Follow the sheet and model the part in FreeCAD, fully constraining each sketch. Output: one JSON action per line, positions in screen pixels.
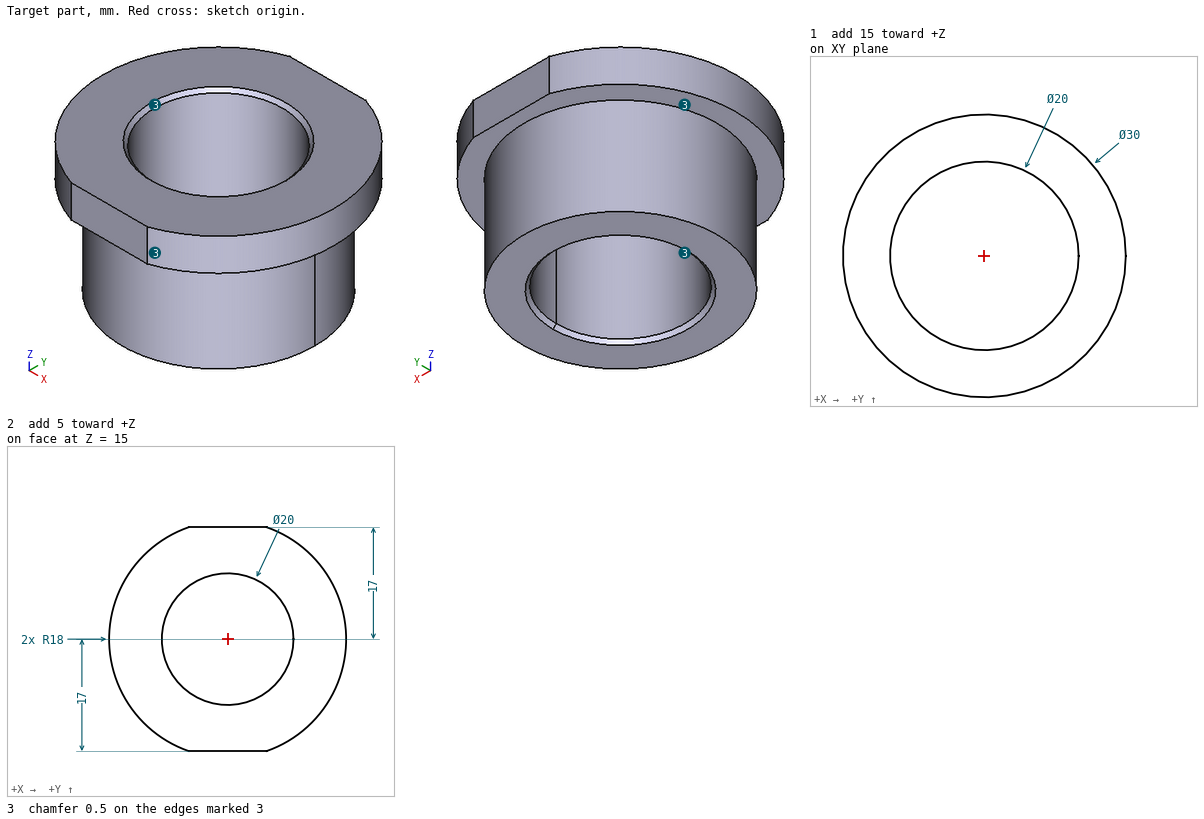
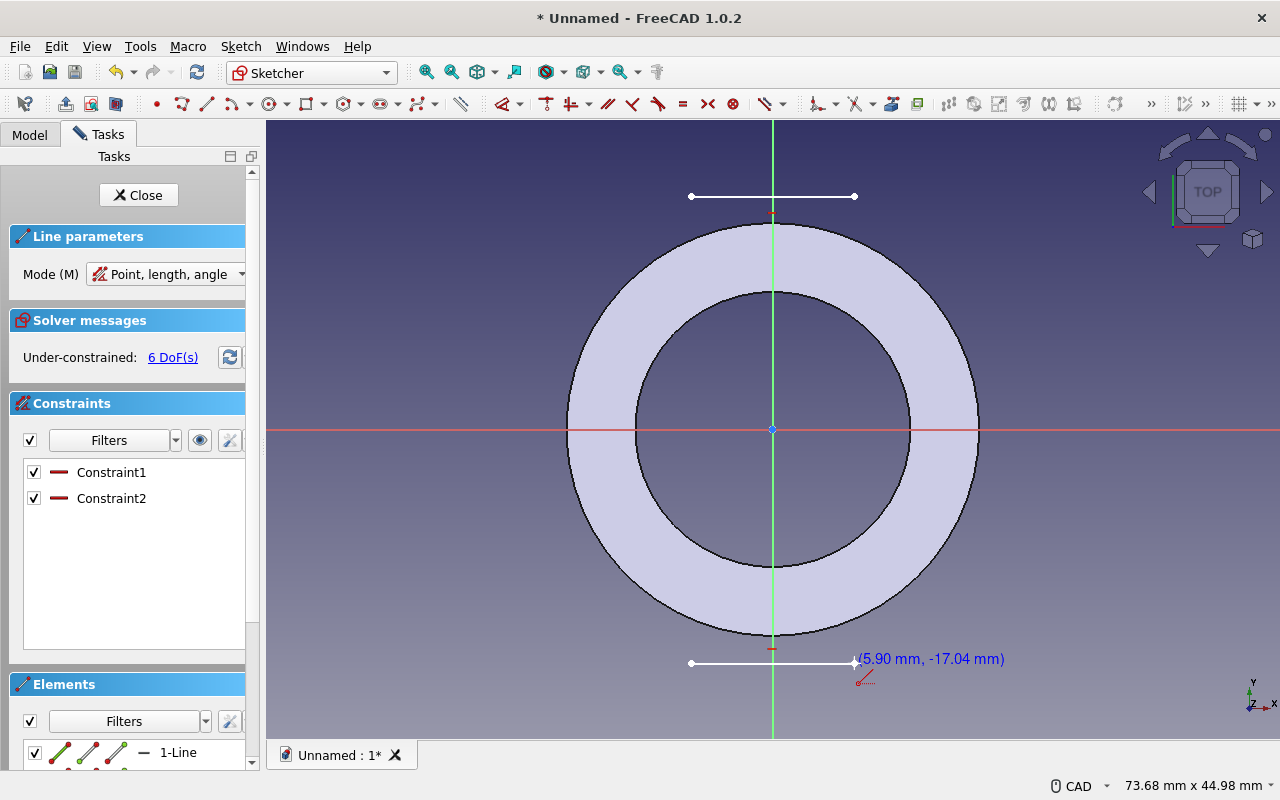
{"action": "left_click", "coordinate": [250, 104]}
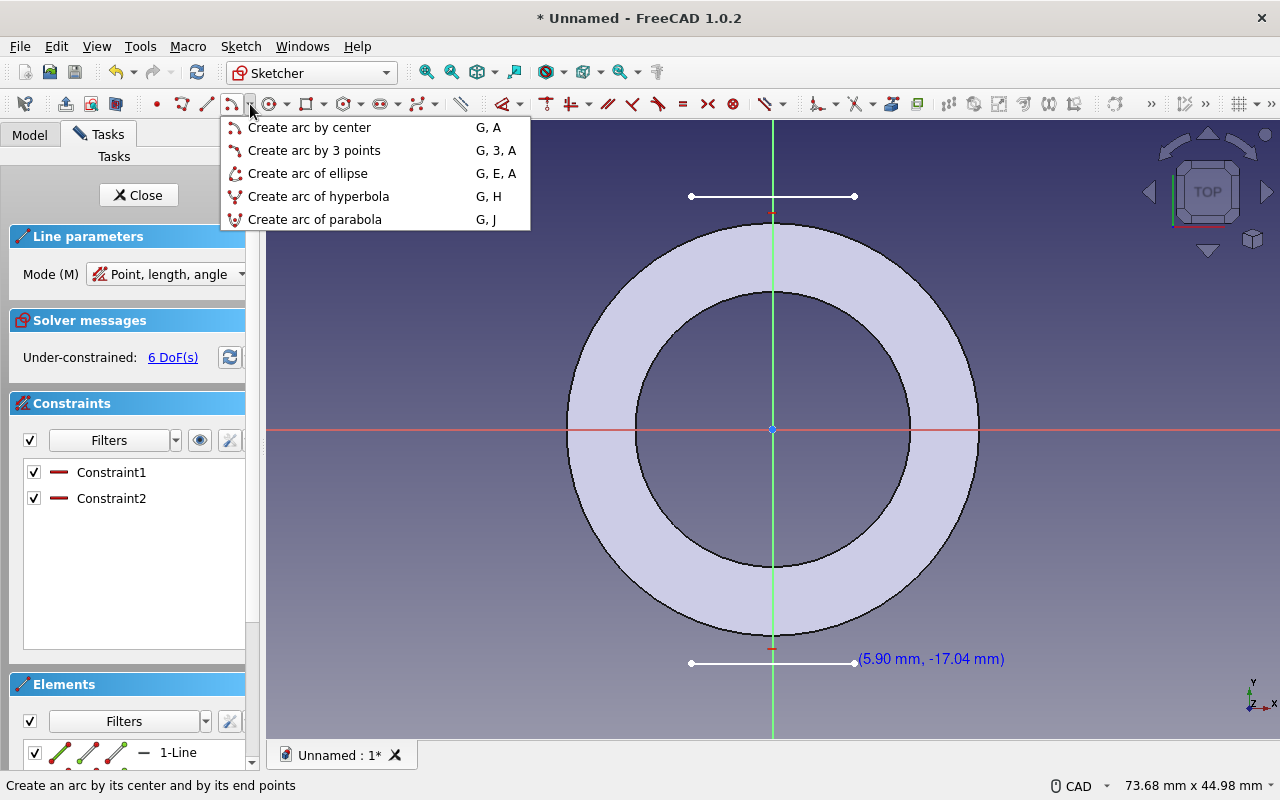
{"action": "left_click", "coordinate": [376, 150]}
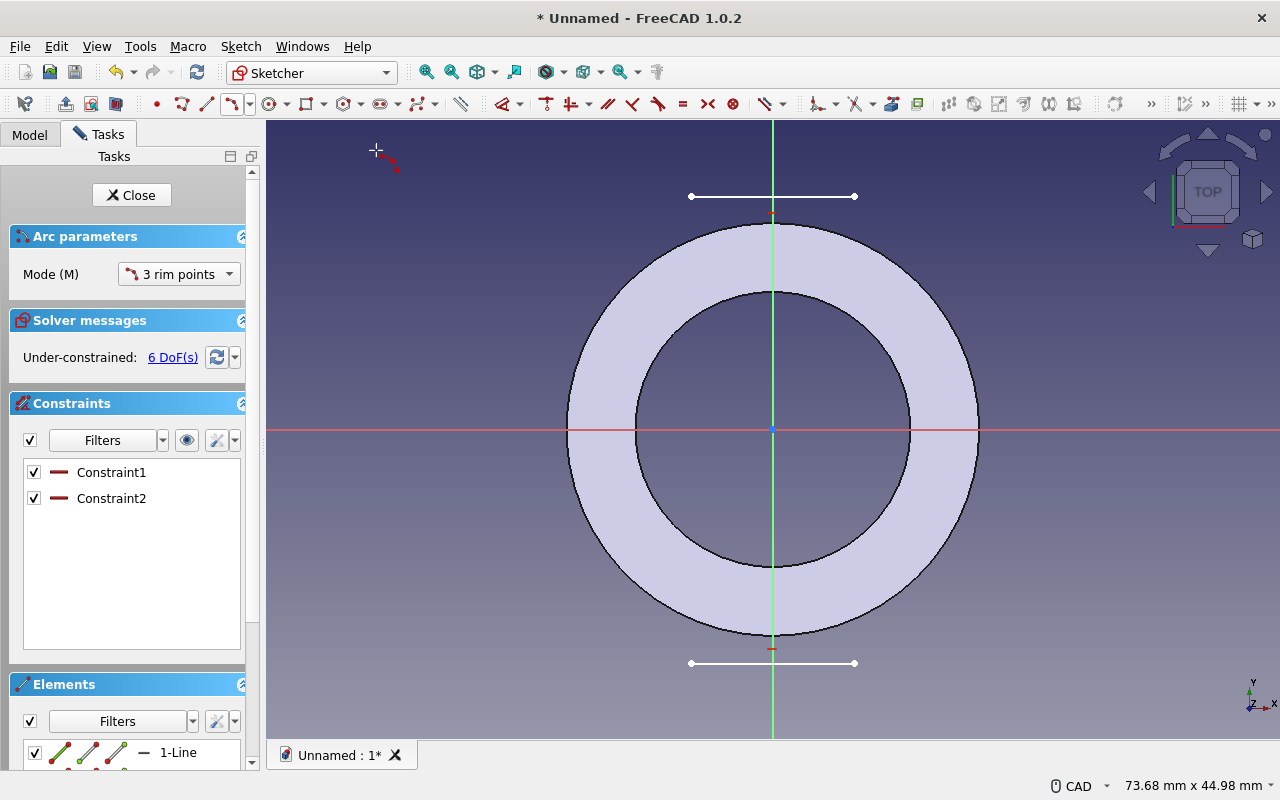
{"action": "left_click", "coordinate": [691, 197]}
{"action": "left_click", "coordinate": [691, 664]}
{"action": "left_click", "coordinate": [533, 369]}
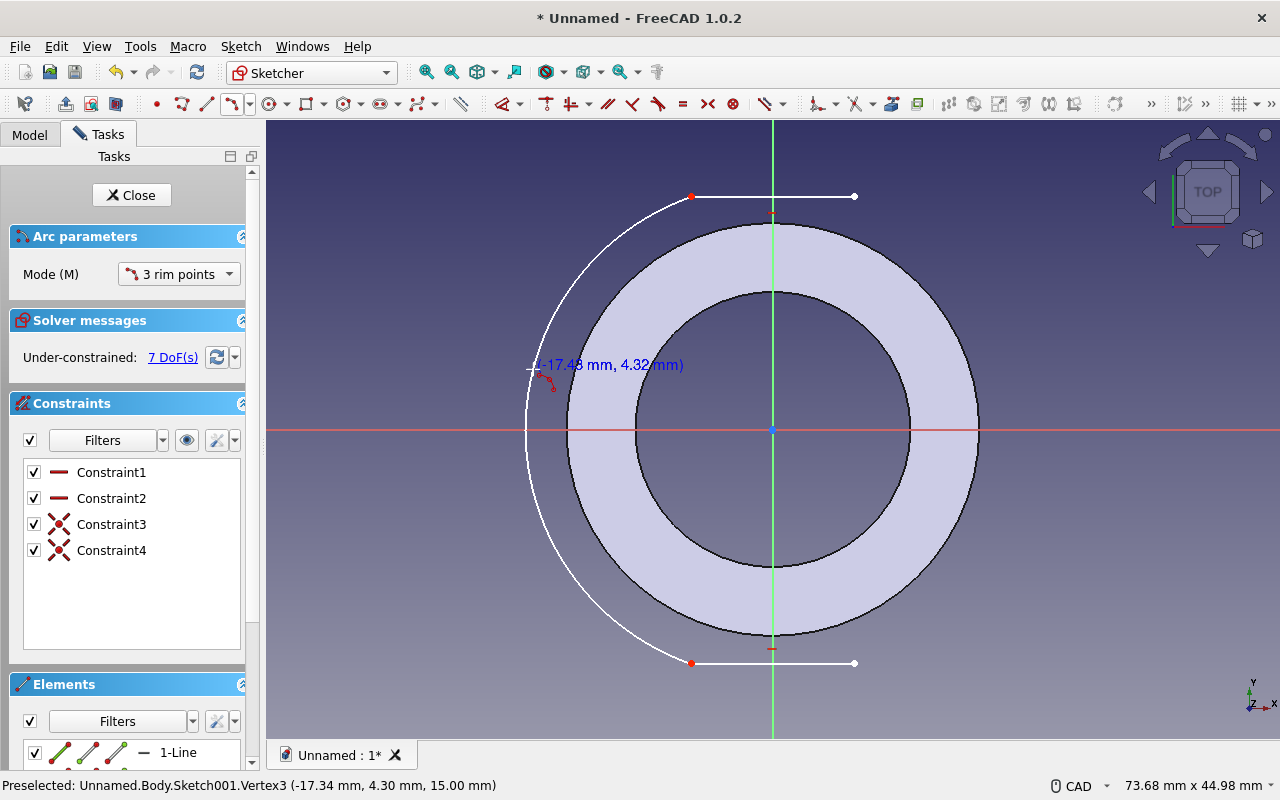
{"action": "left_click", "coordinate": [854, 664]}
{"action": "left_click", "coordinate": [854, 197]}
{"action": "left_click", "coordinate": [1013, 490]}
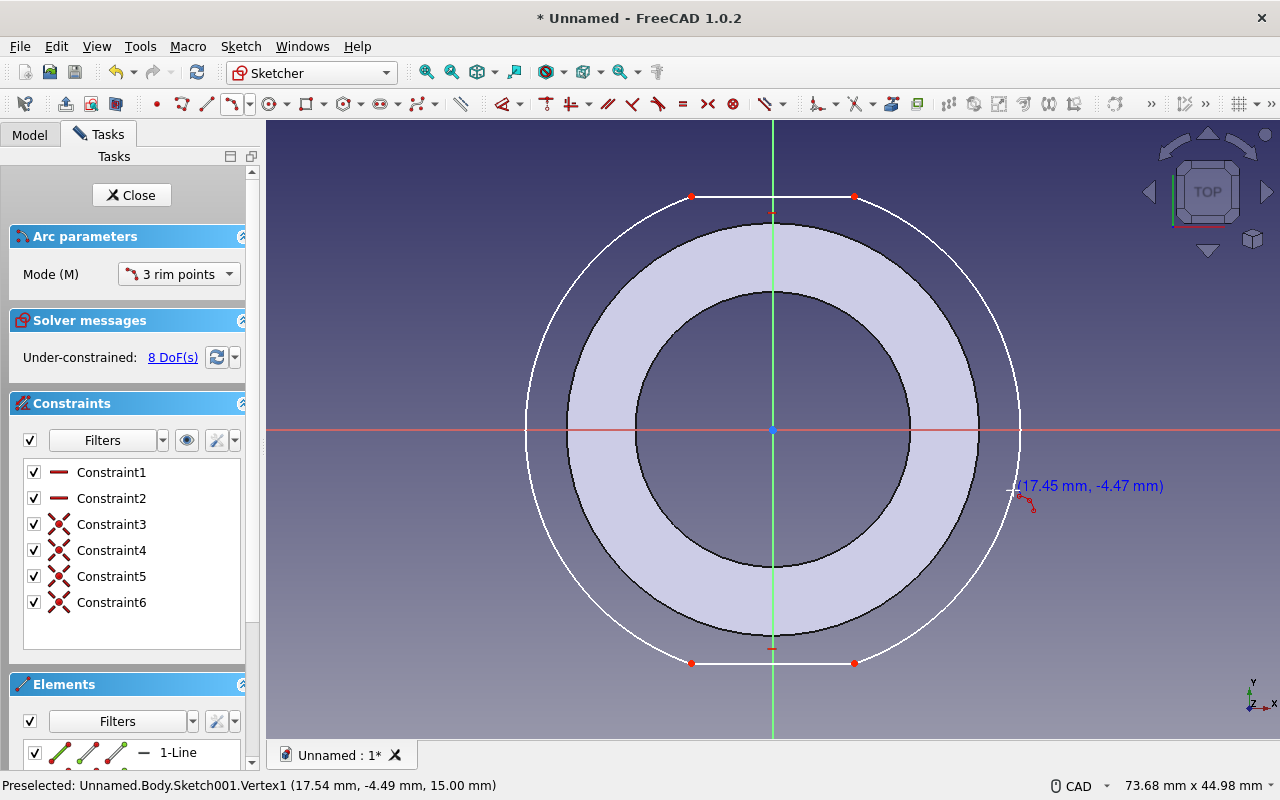
{"action": "left_click", "coordinate": [268, 104]}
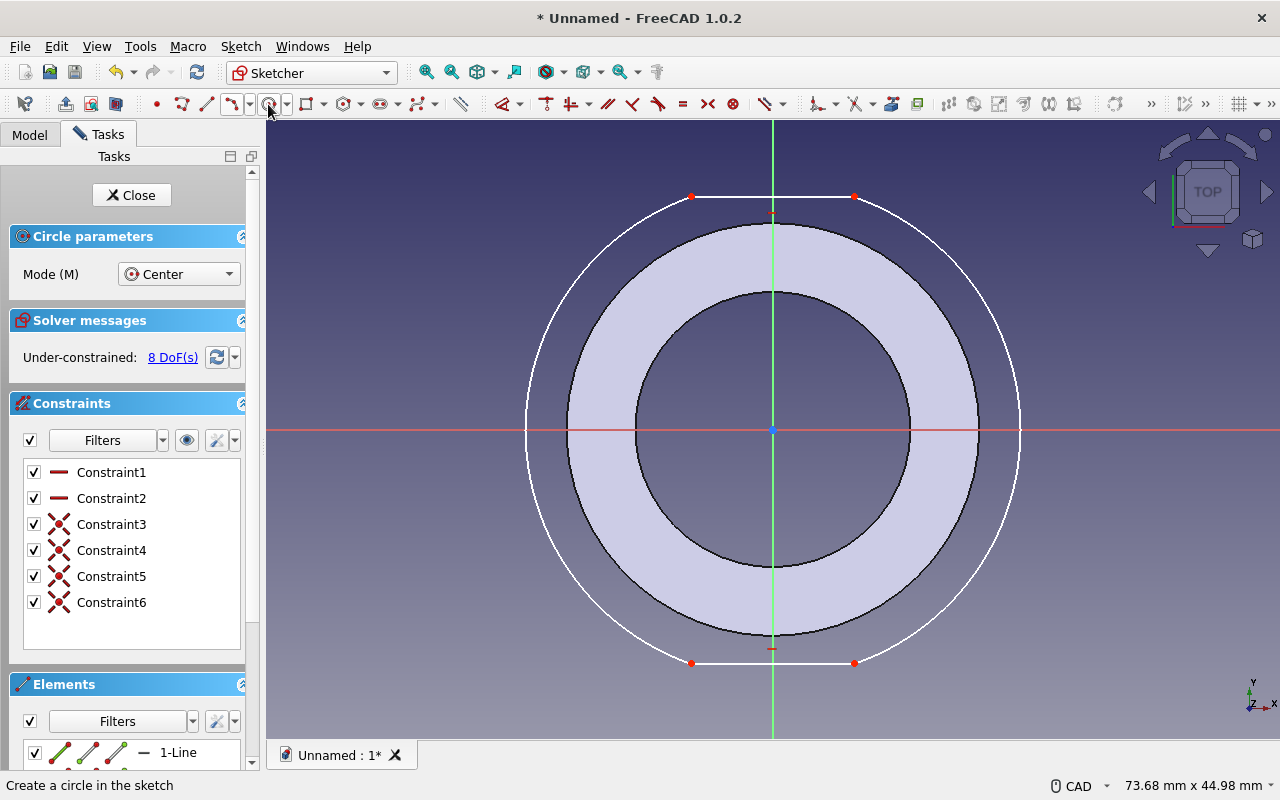
{"action": "left_click", "coordinate": [773, 430]}
{"action": "mouse_move", "coordinate": [870, 332]}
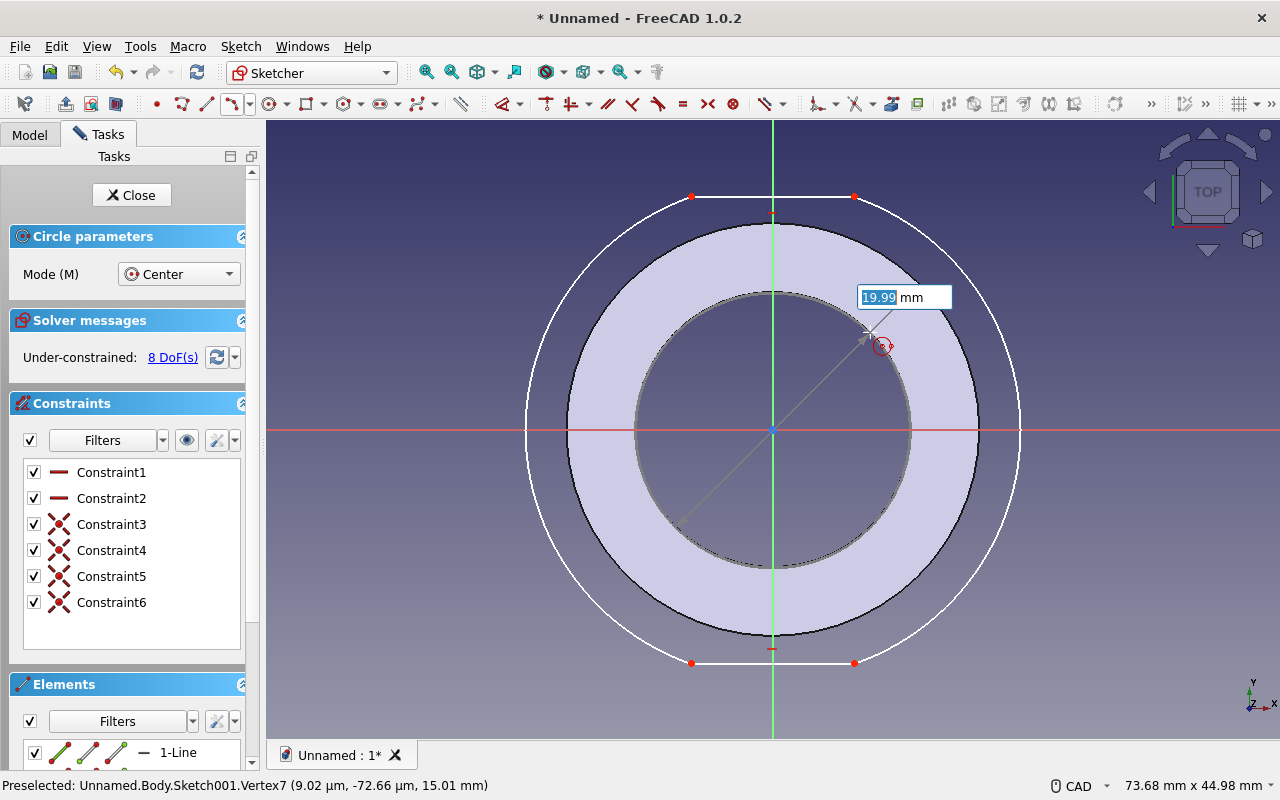
{"action": "type", "text": "20"}
{"action": "key", "text": "Return"}
{"action": "key", "text": "Escape"}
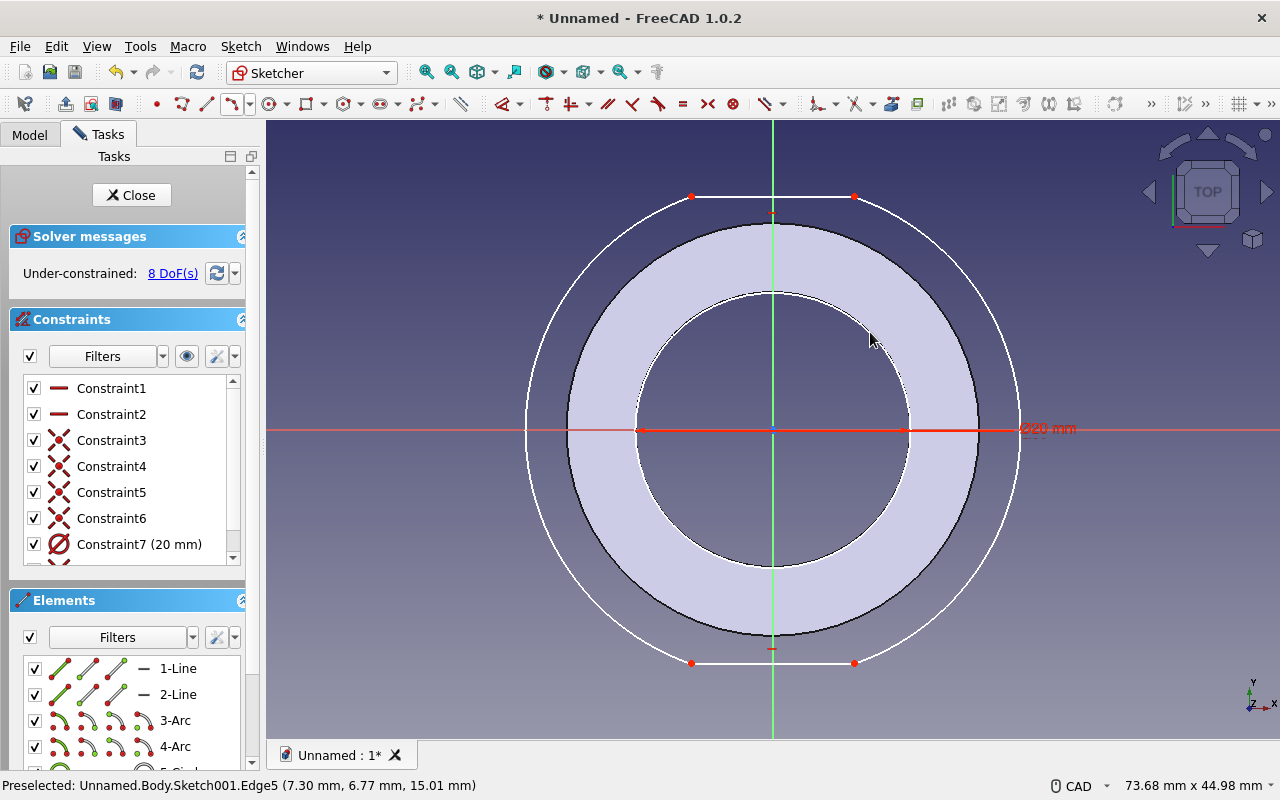
{"action": "left_click", "coordinate": [870, 333]}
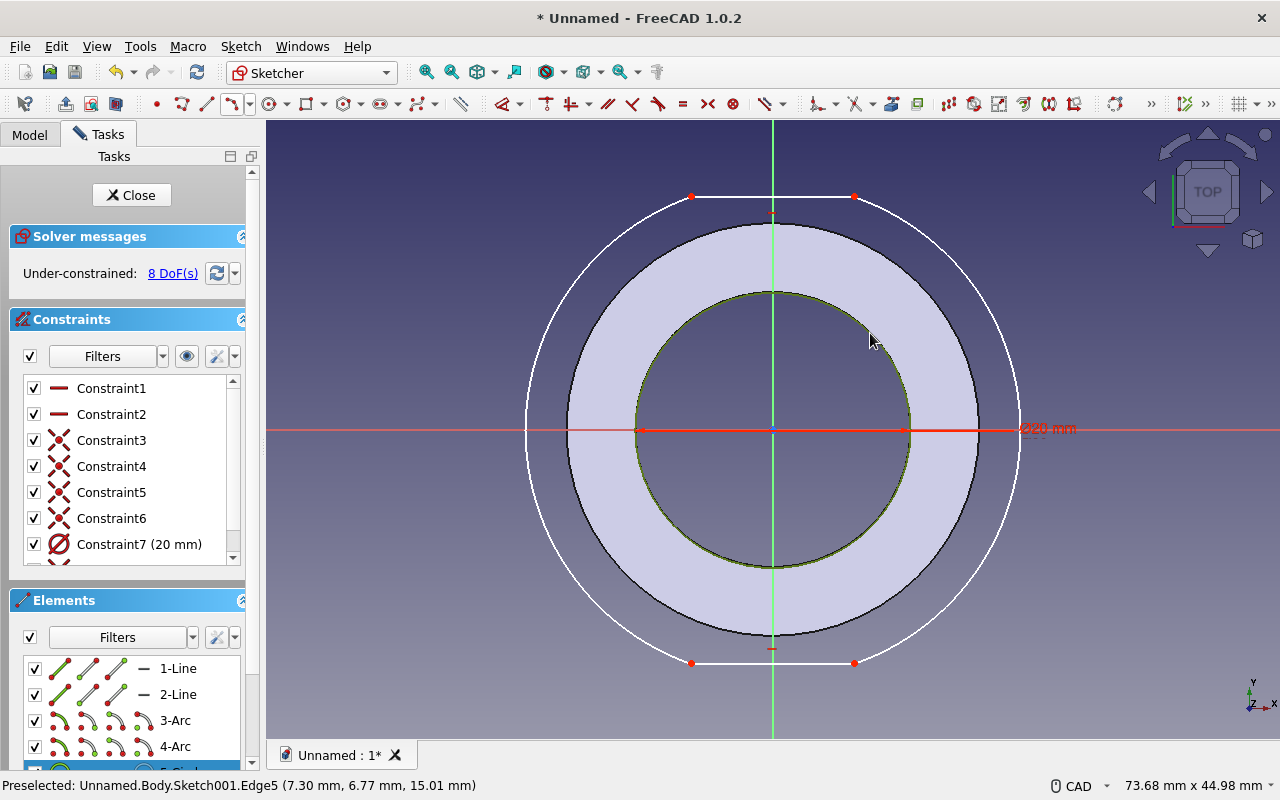
{"action": "left_click", "coordinate": [991, 548]}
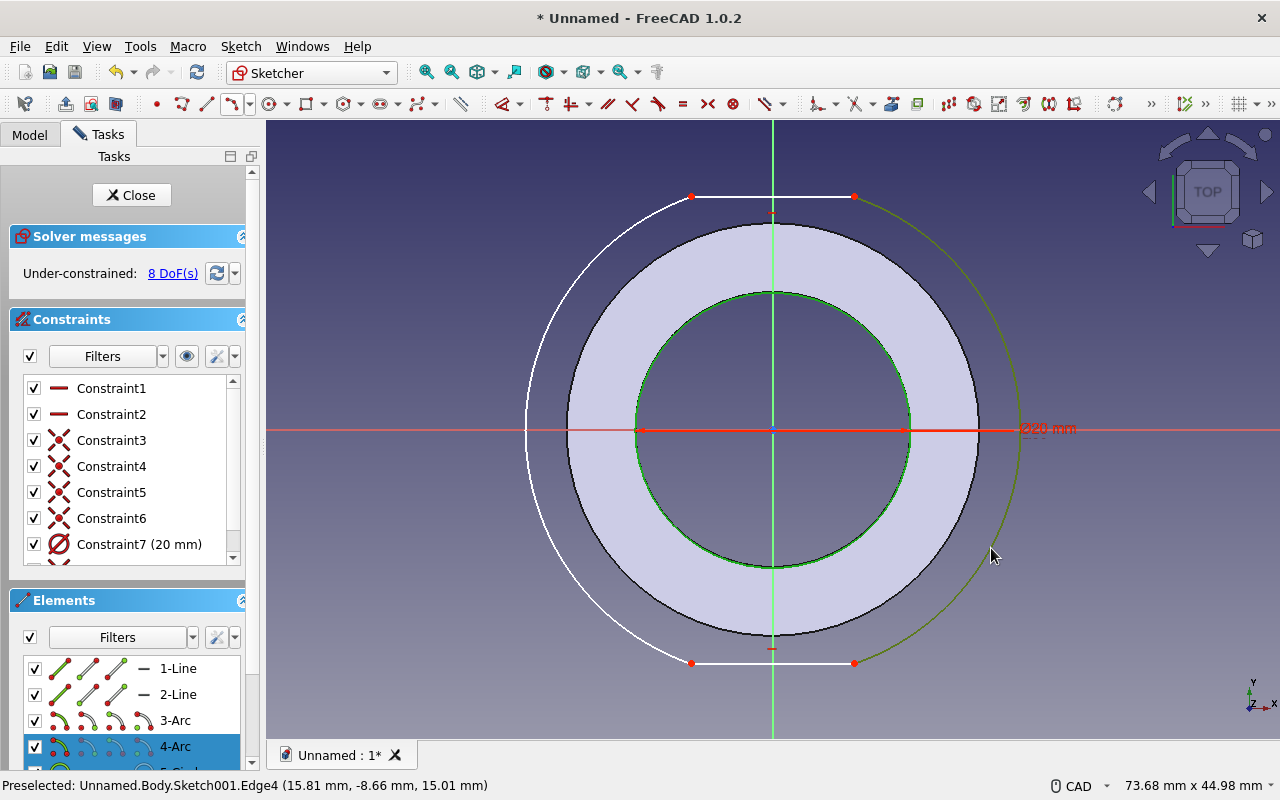
{"action": "left_click", "coordinate": [546, 104]}